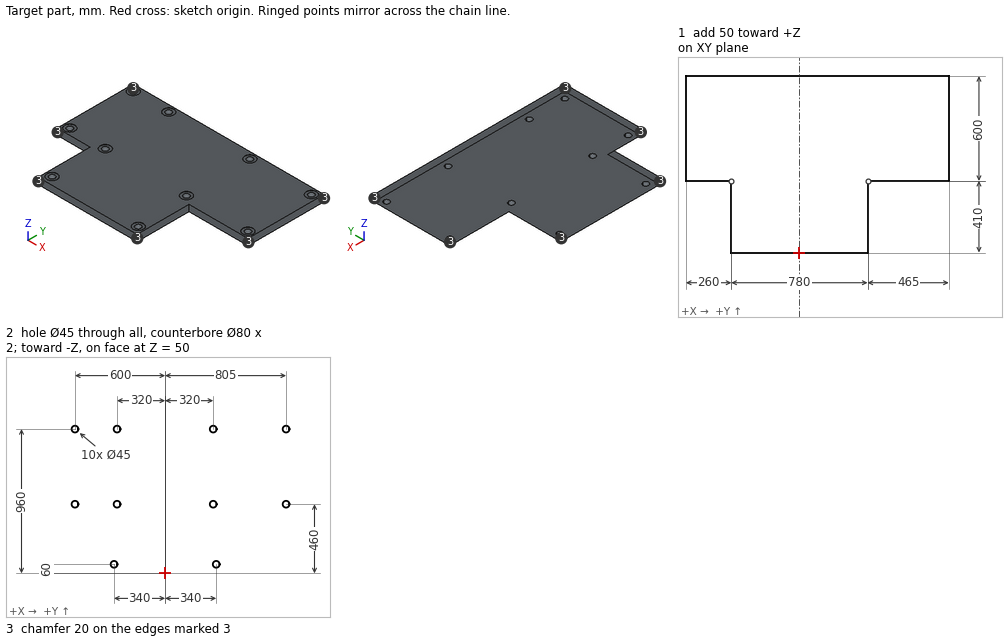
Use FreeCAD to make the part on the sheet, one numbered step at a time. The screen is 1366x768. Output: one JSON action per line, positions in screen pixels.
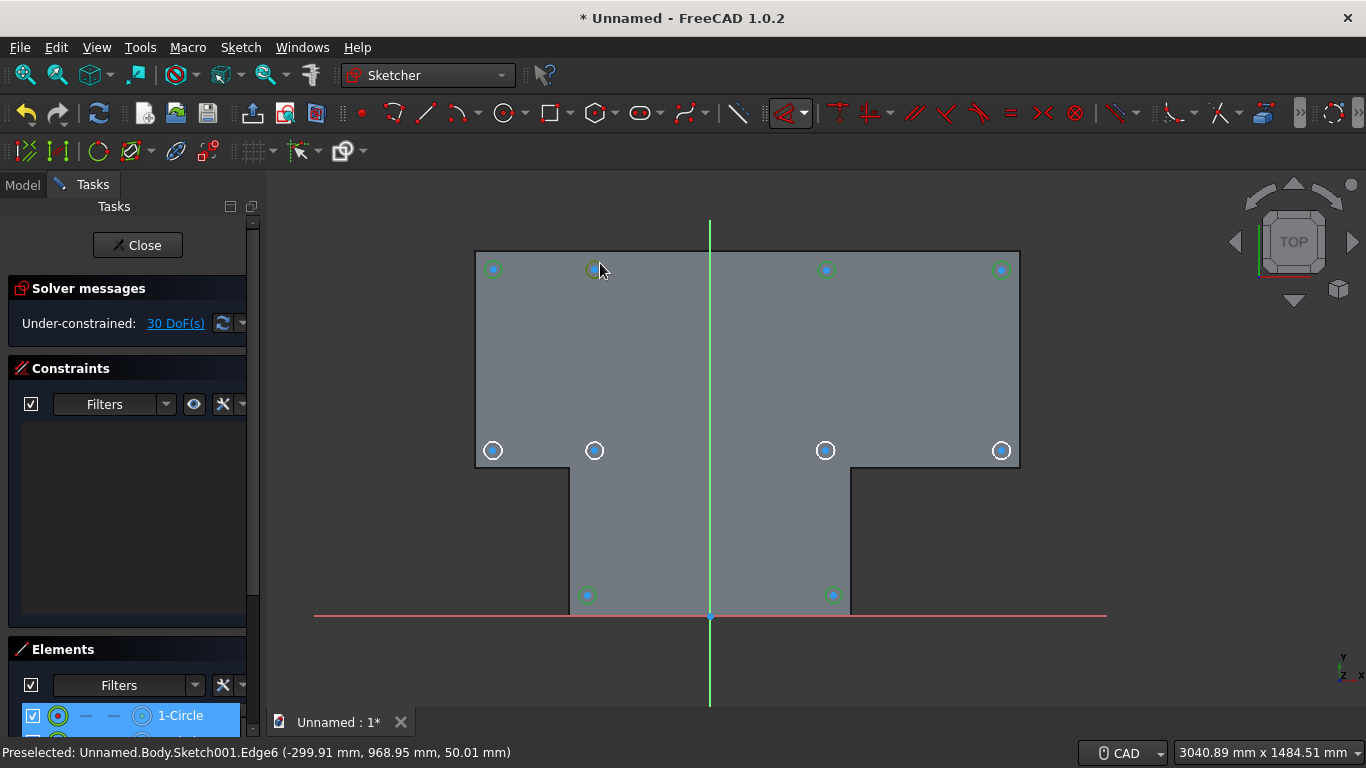
{"action": "scroll", "coordinate": [1008, 445], "scroll_direction": "up", "scroll_amount": 3}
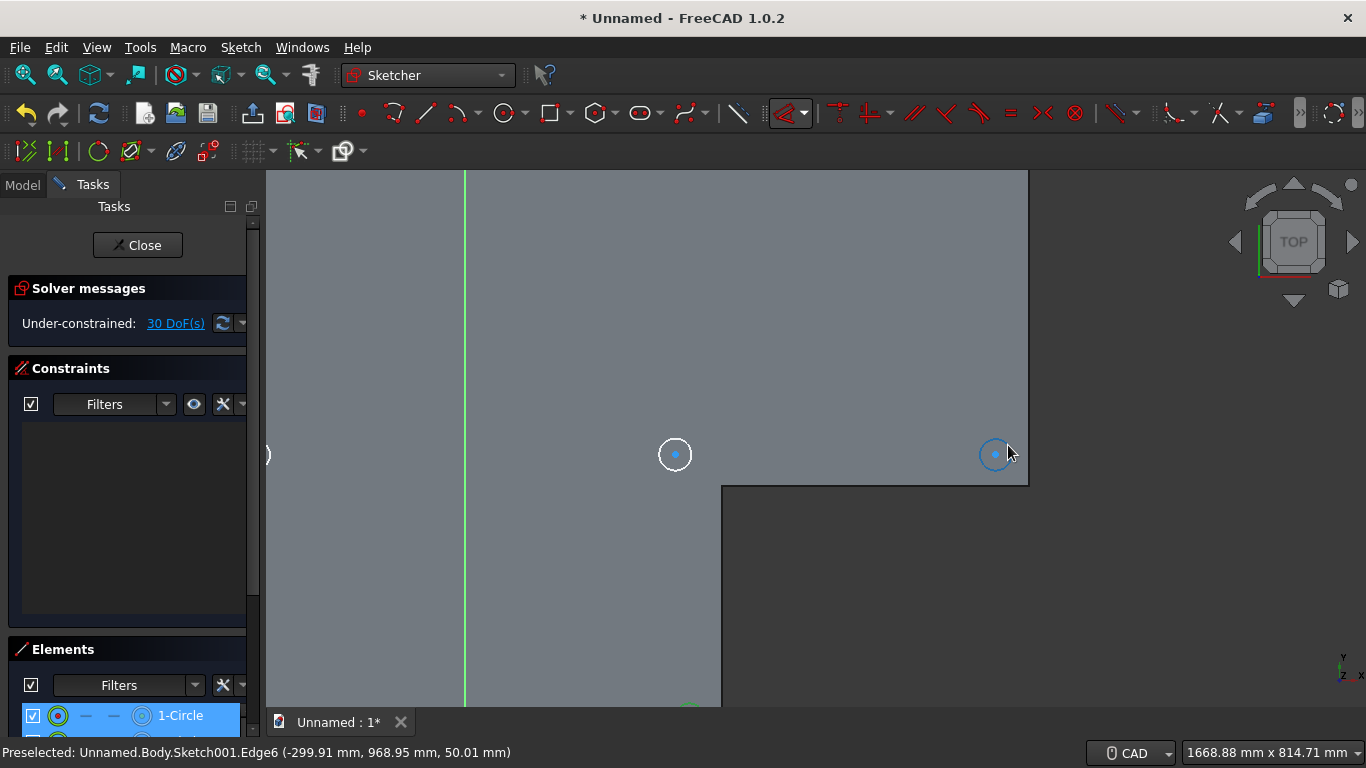
{"action": "left_click", "coordinate": [1007, 444]}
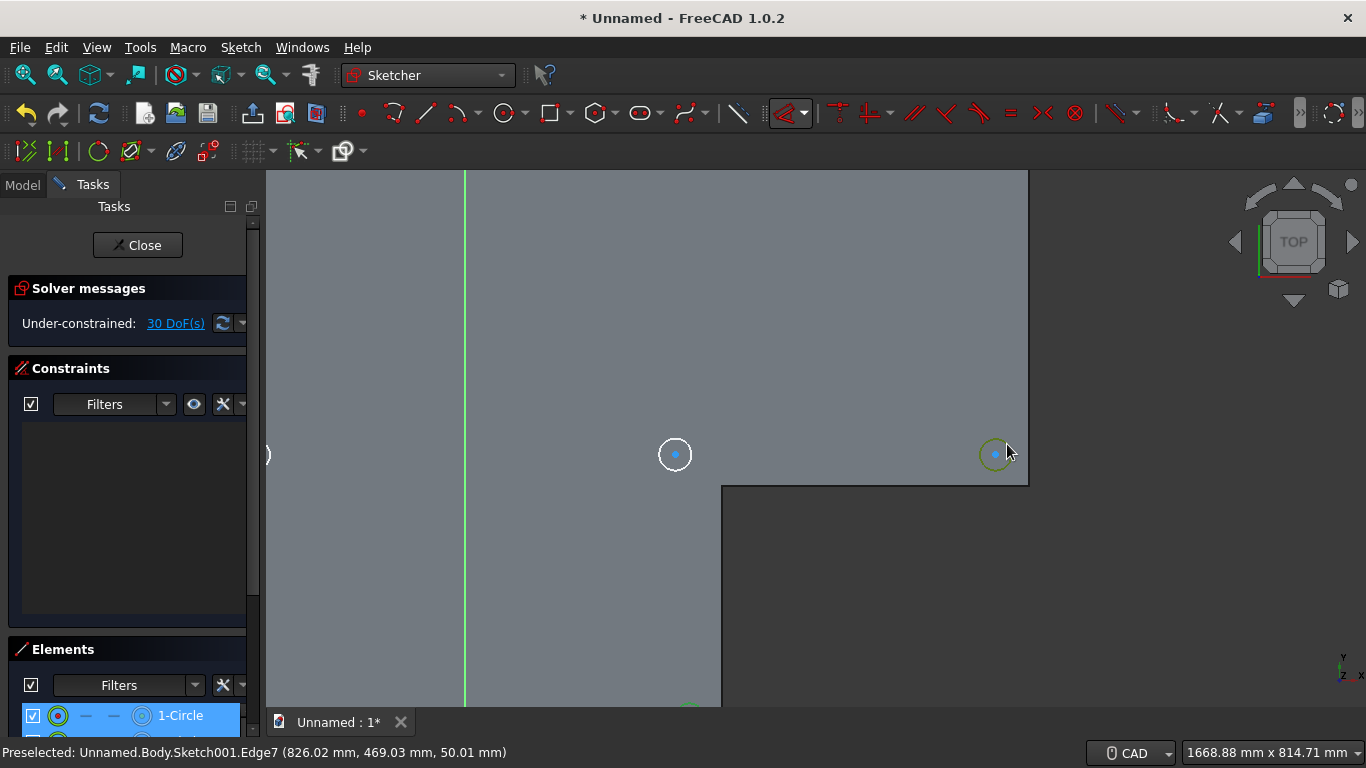
{"action": "left_click", "coordinate": [687, 443]}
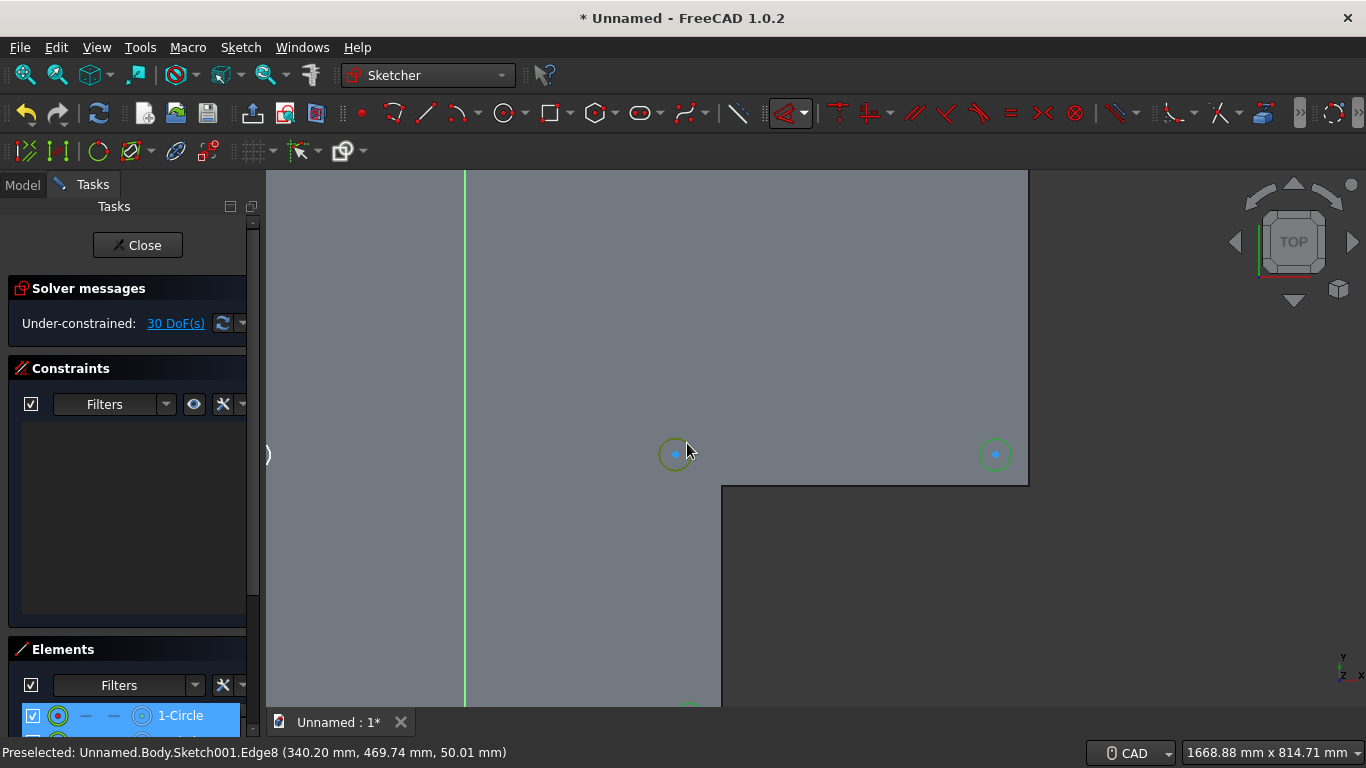
{"action": "scroll", "coordinate": [1009, 446], "scroll_direction": "down", "scroll_amount": 3}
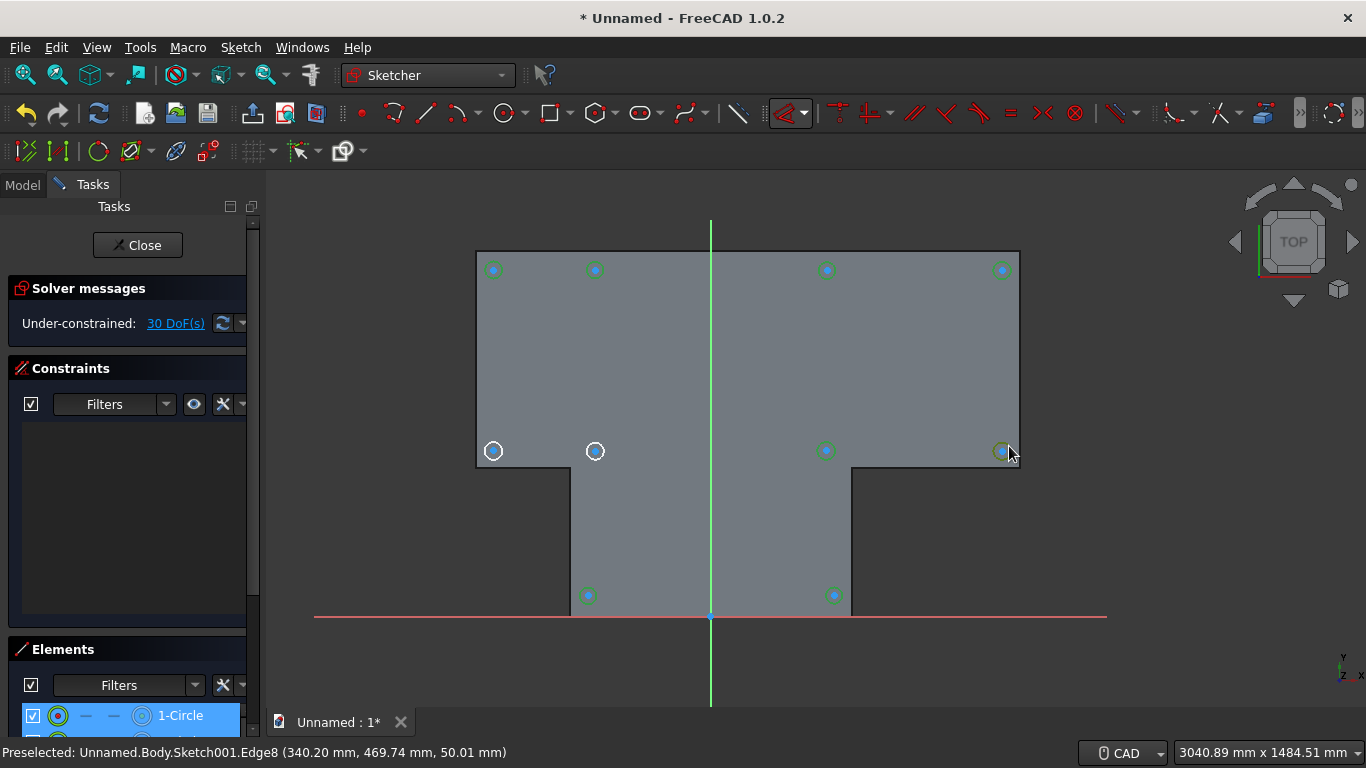
{"action": "scroll", "coordinate": [601, 445], "scroll_direction": "up", "scroll_amount": 3}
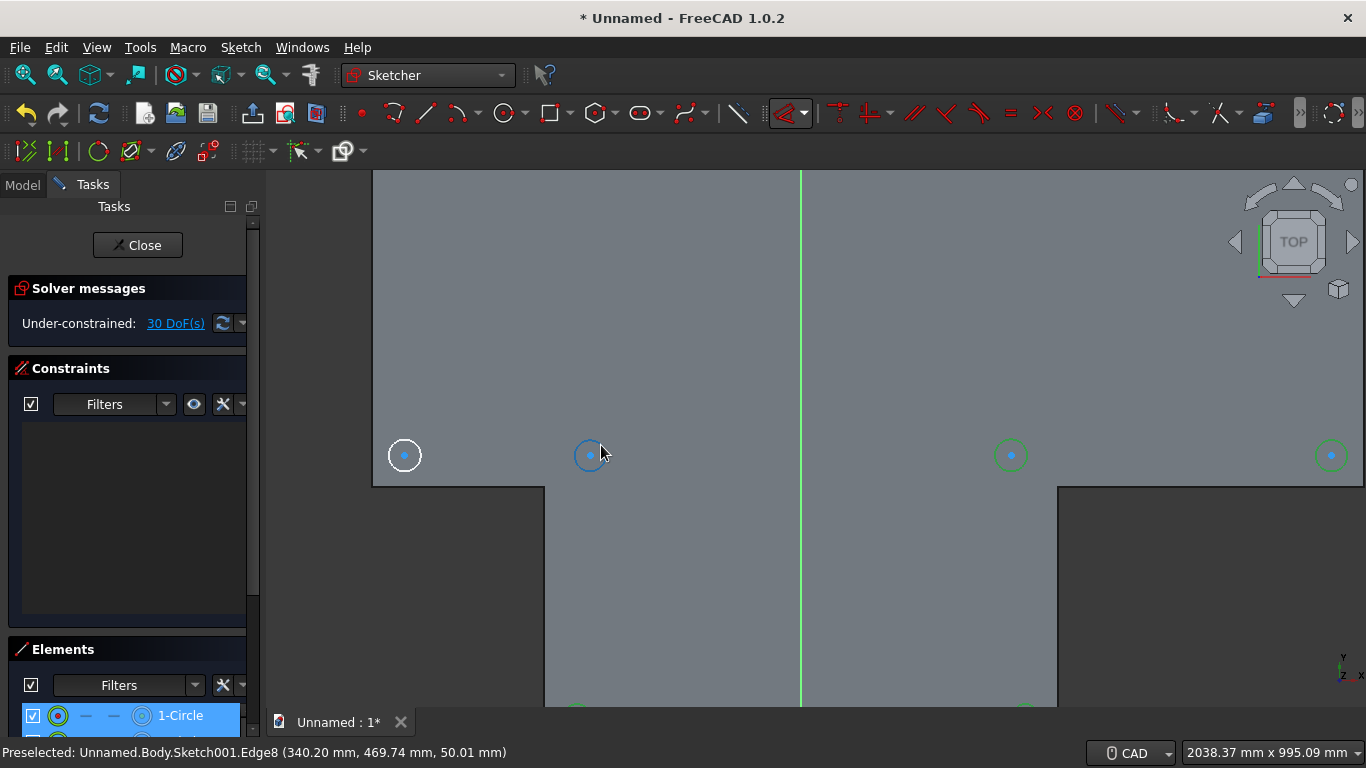
{"action": "left_click", "coordinate": [601, 445]}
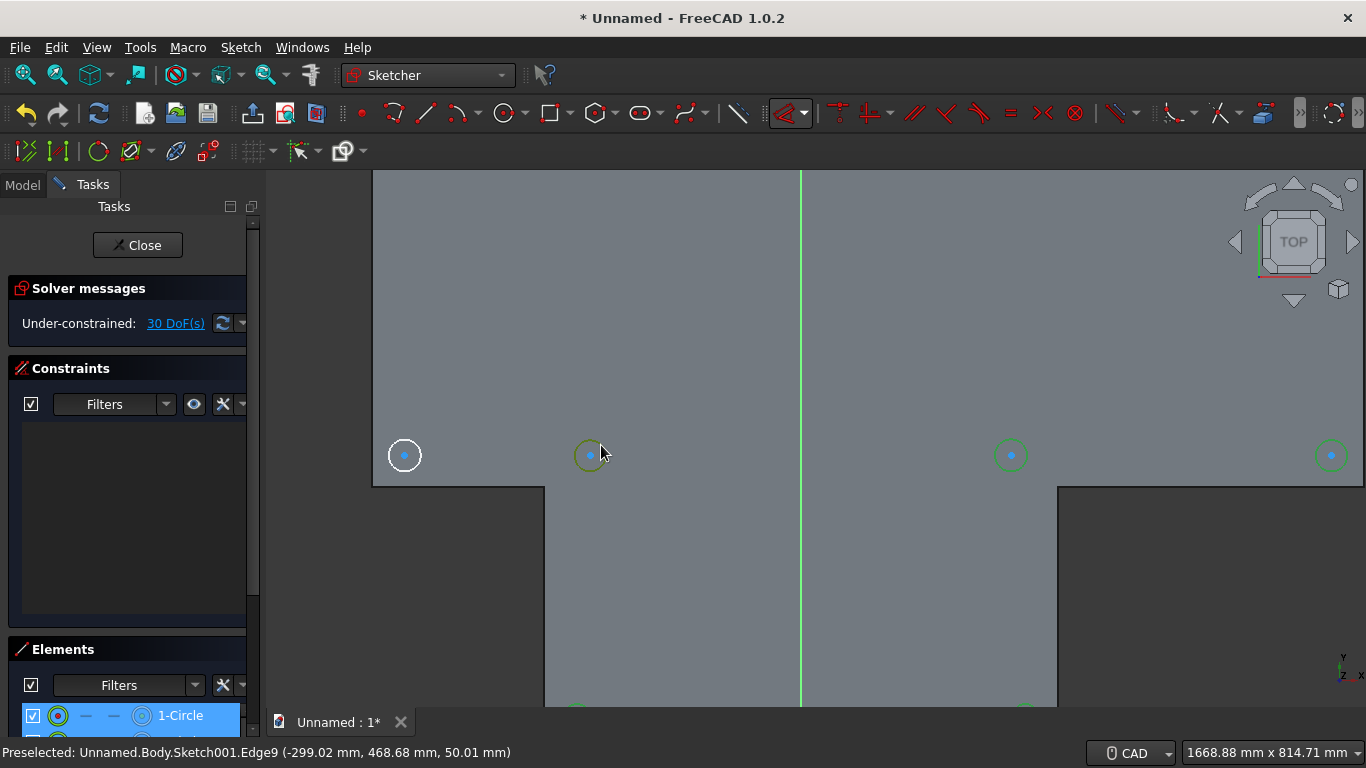
{"action": "left_click", "coordinate": [416, 444]}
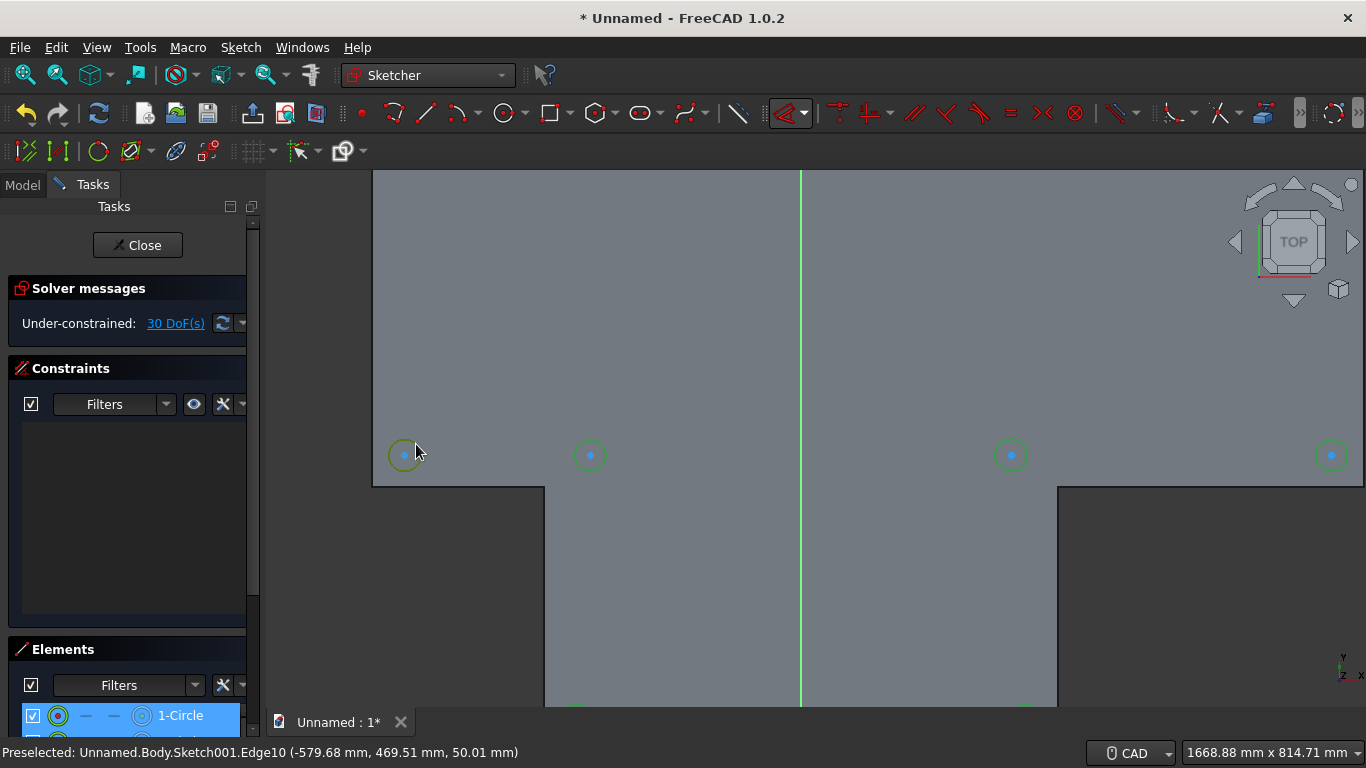
{"action": "left_click", "coordinate": [1012, 114]}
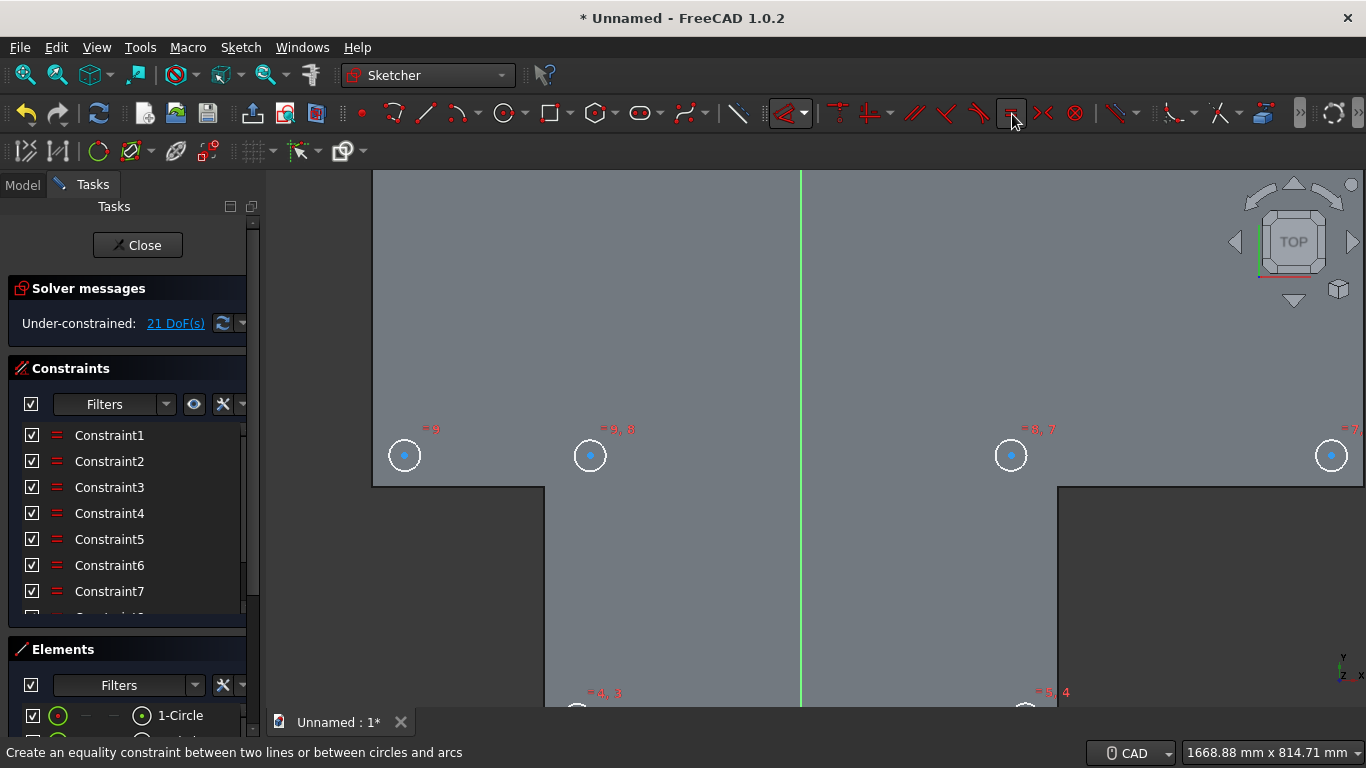
{"action": "scroll", "coordinate": [600, 445], "scroll_direction": "down", "scroll_amount": 3}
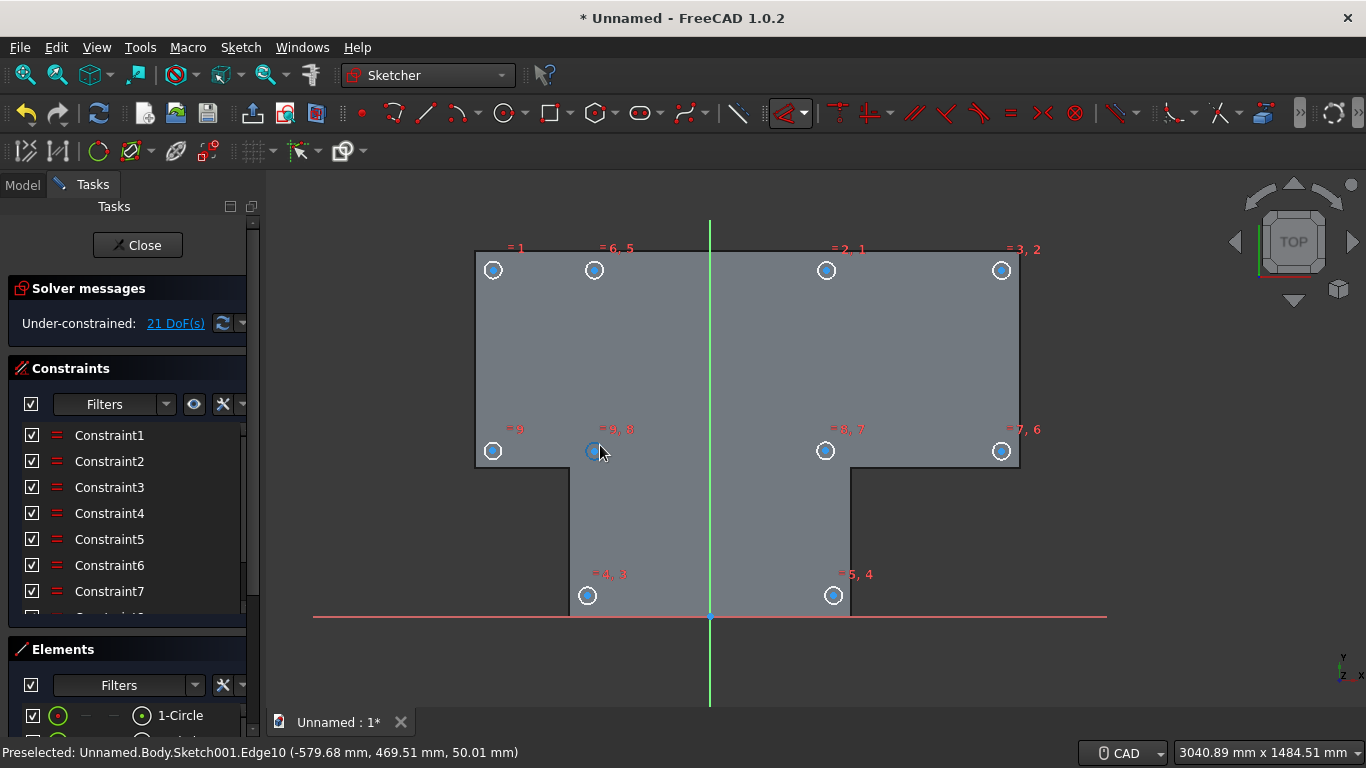
{"action": "left_click", "coordinate": [493, 270]}